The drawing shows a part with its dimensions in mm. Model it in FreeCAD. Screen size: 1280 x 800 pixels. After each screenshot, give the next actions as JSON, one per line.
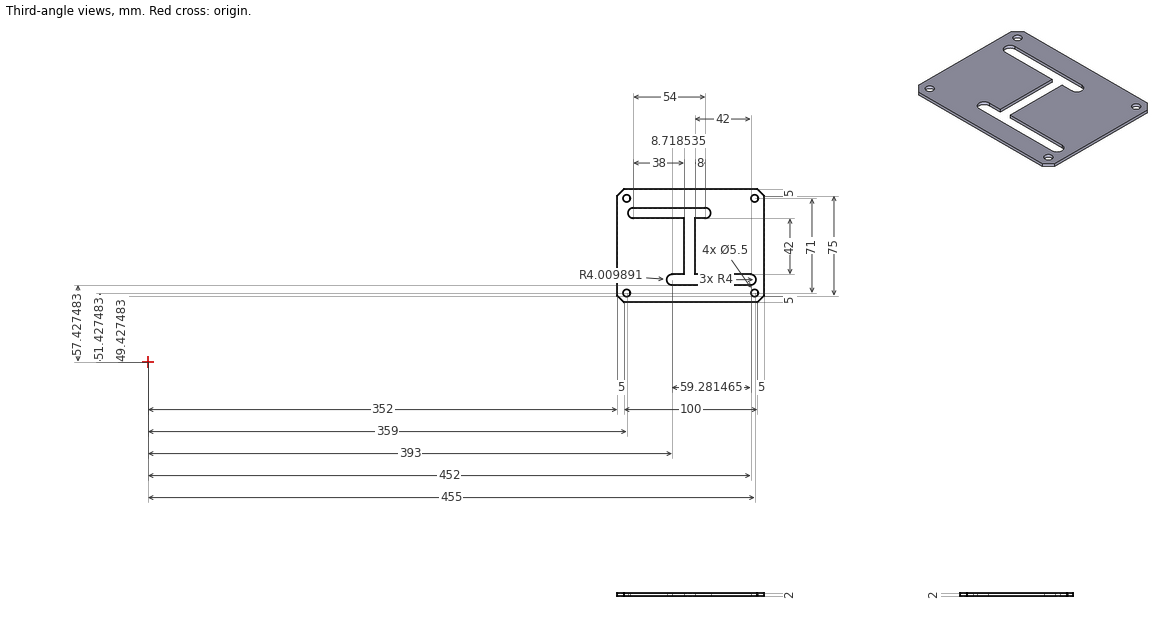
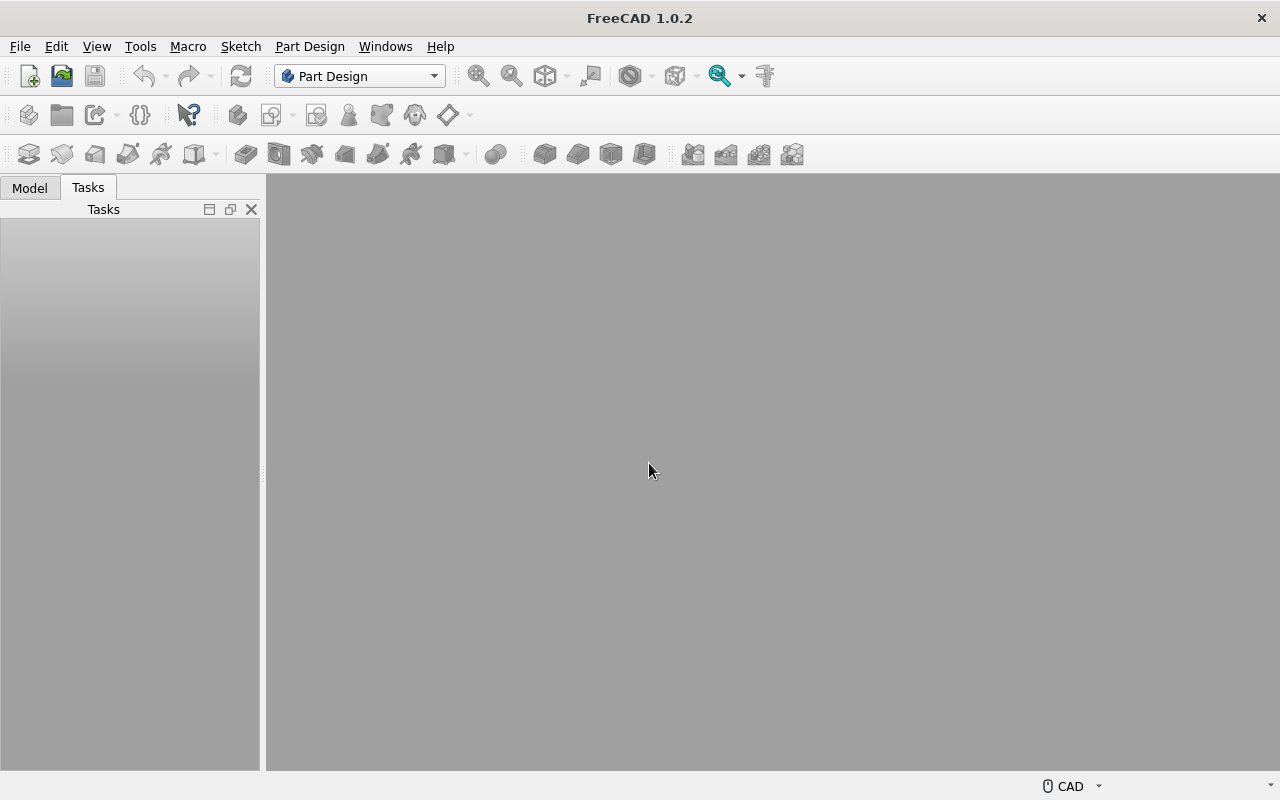
{"action": "left_click", "coordinate": [29, 76]}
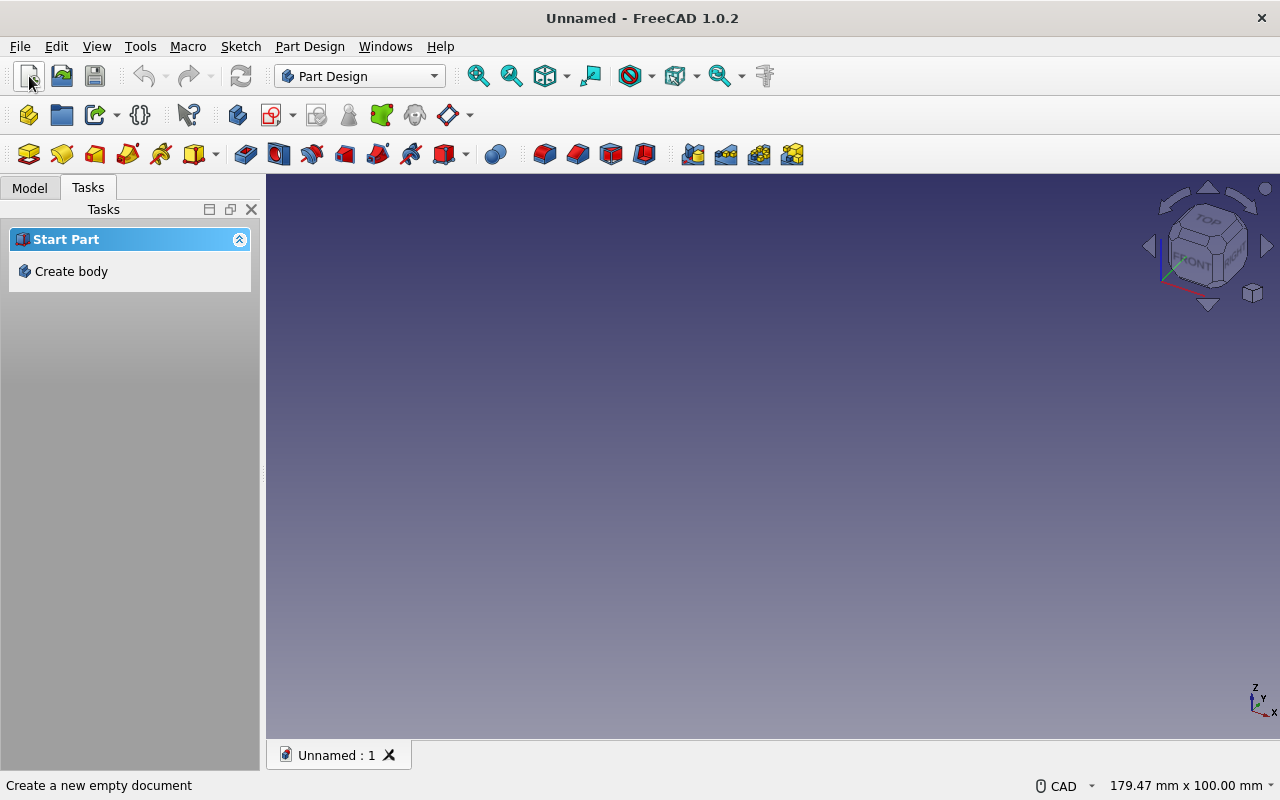
{"action": "left_click", "coordinate": [270, 116]}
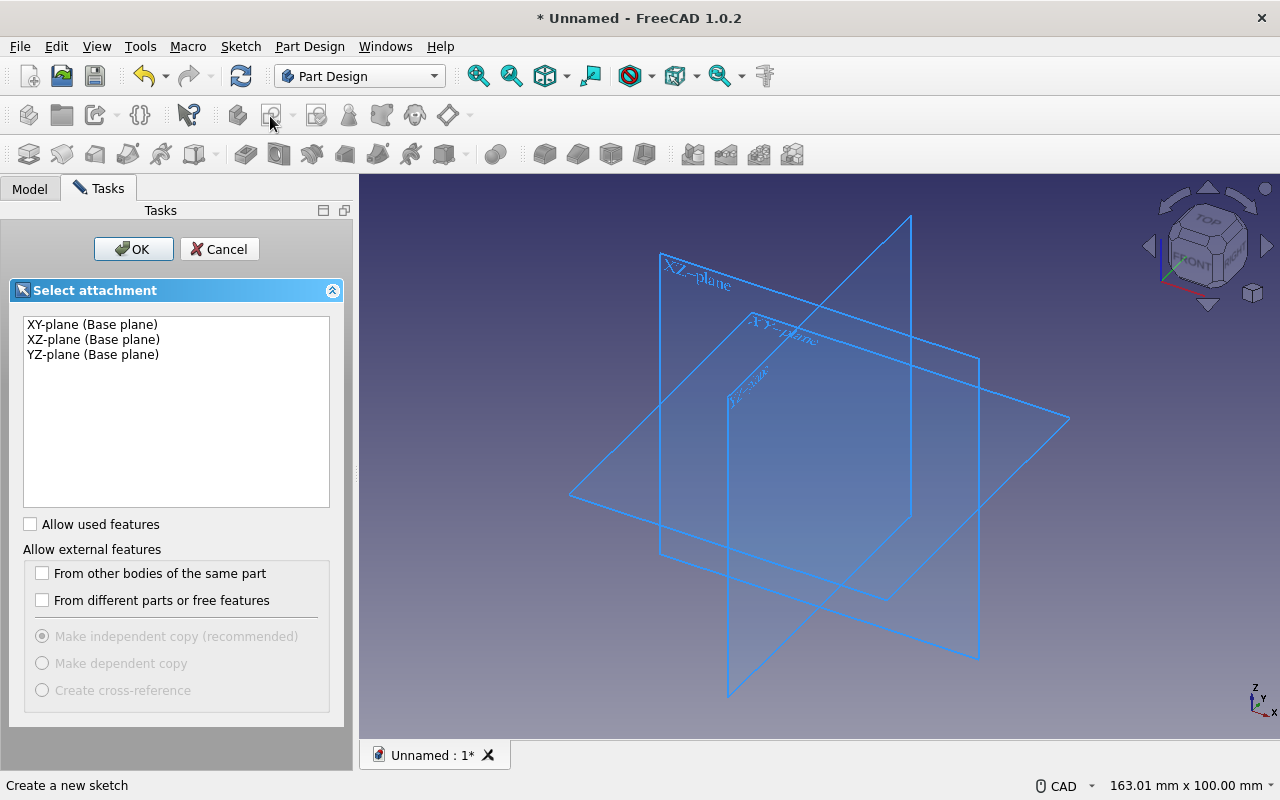
{"action": "left_click", "coordinate": [84, 324]}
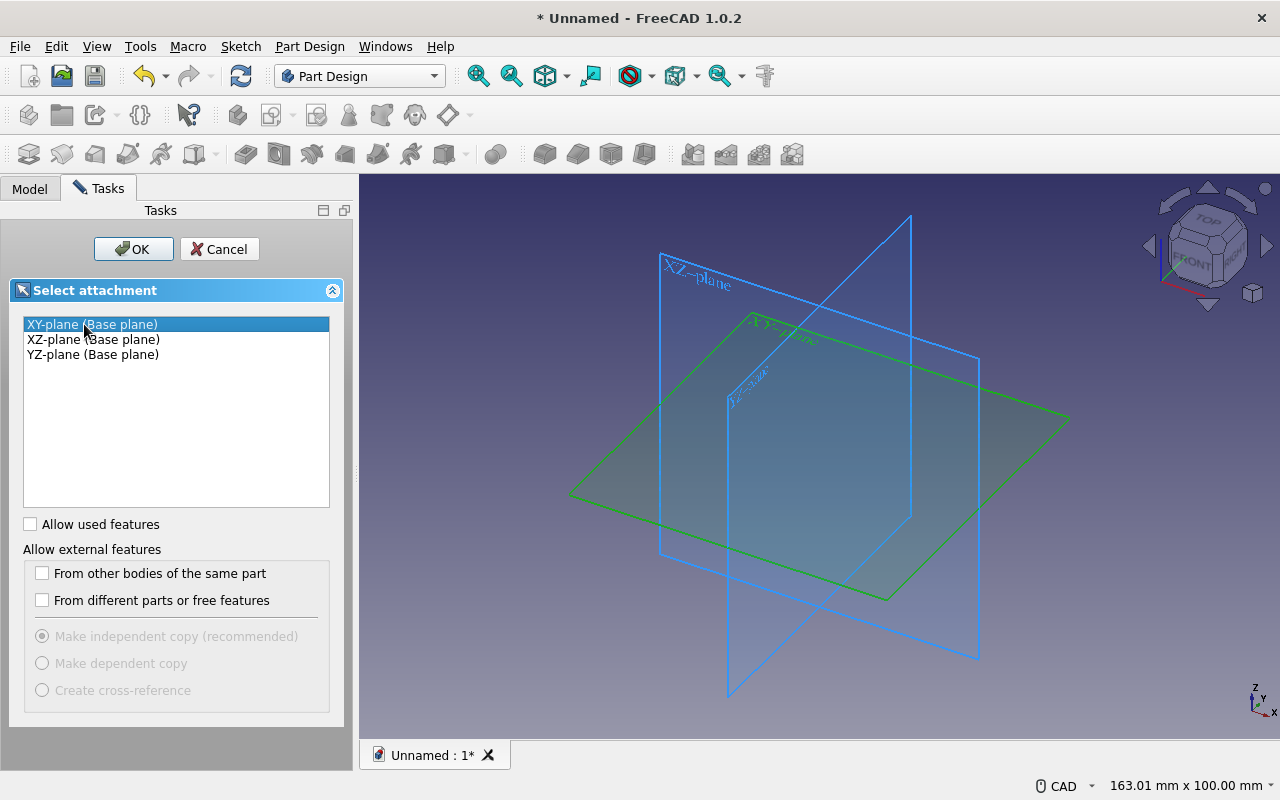
{"action": "left_click", "coordinate": [134, 249]}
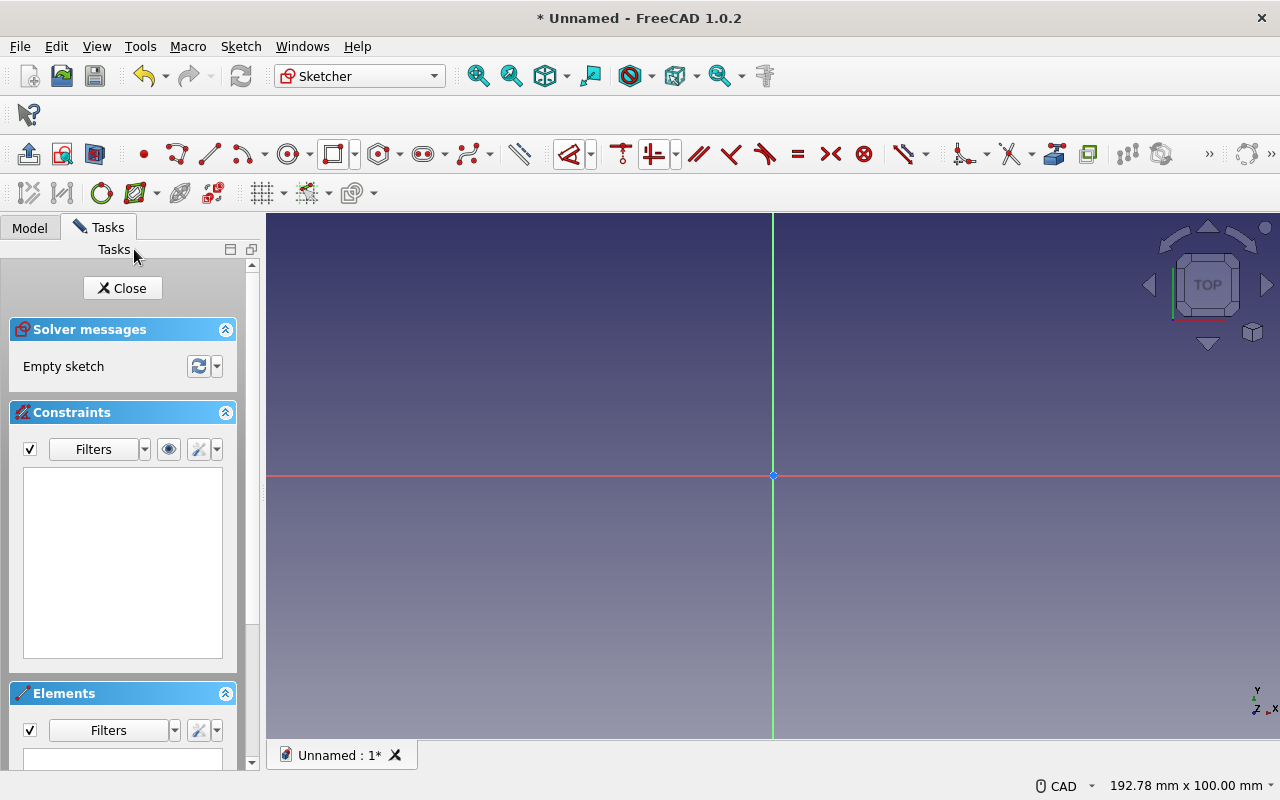
{"action": "scroll", "coordinate": [704, 476], "scroll_direction": "down", "scroll_amount": 5}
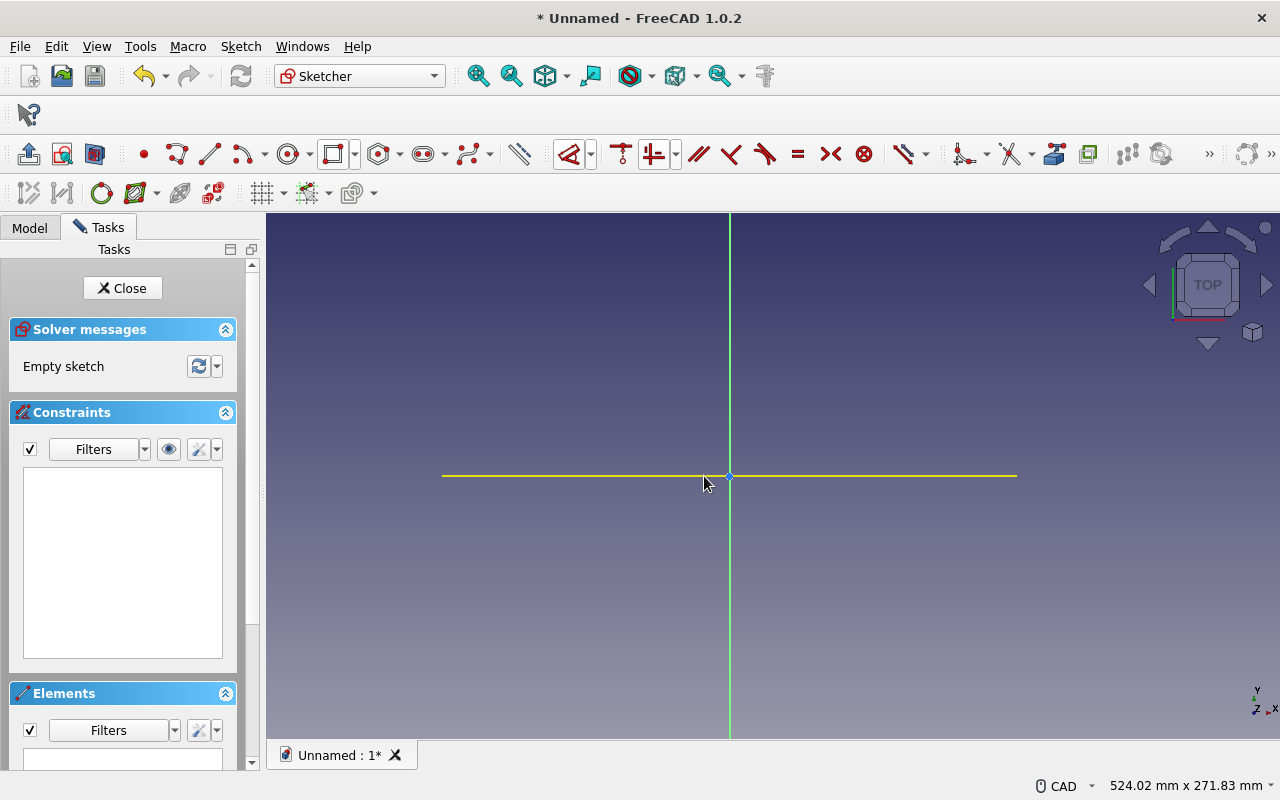
{"action": "scroll", "coordinate": [704, 476], "scroll_direction": "down", "scroll_amount": 5}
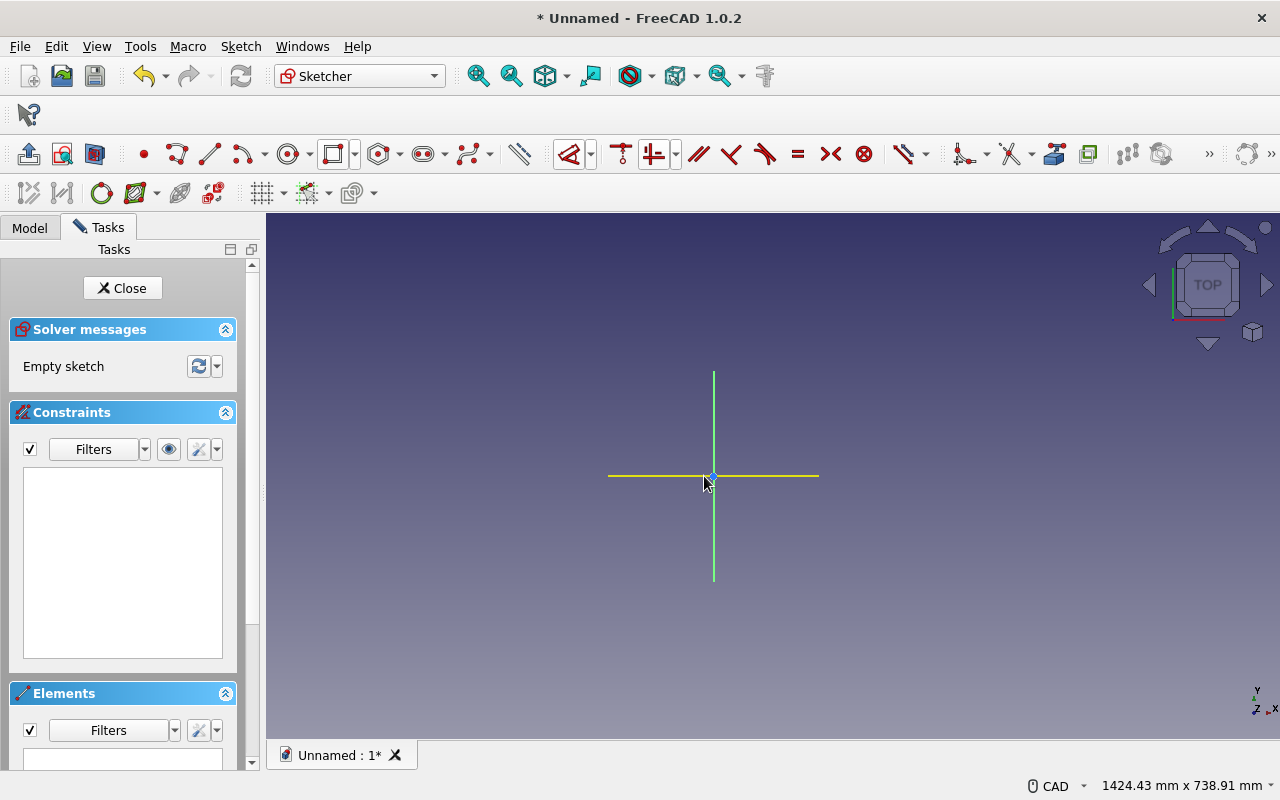
{"action": "scroll", "coordinate": [1063, 402], "scroll_direction": "up", "scroll_amount": 9}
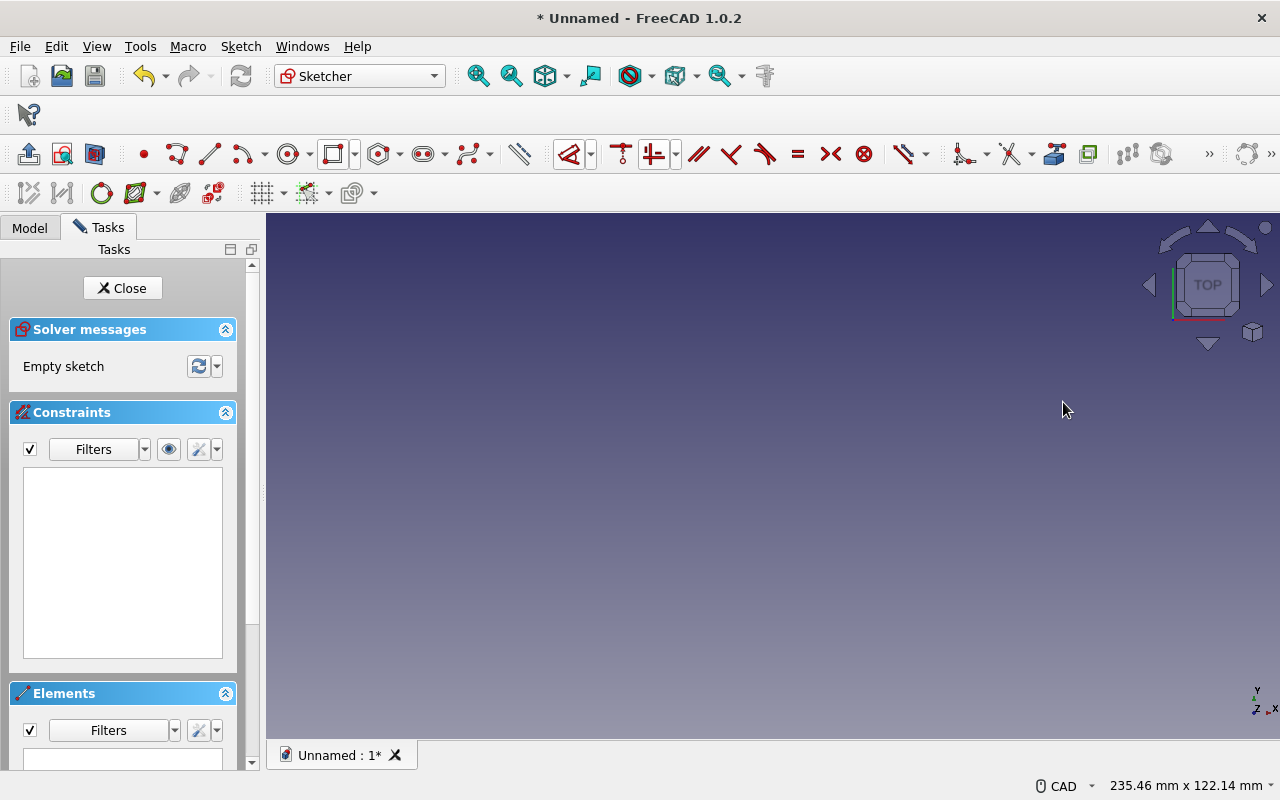
{"action": "left_click", "coordinate": [177, 154]}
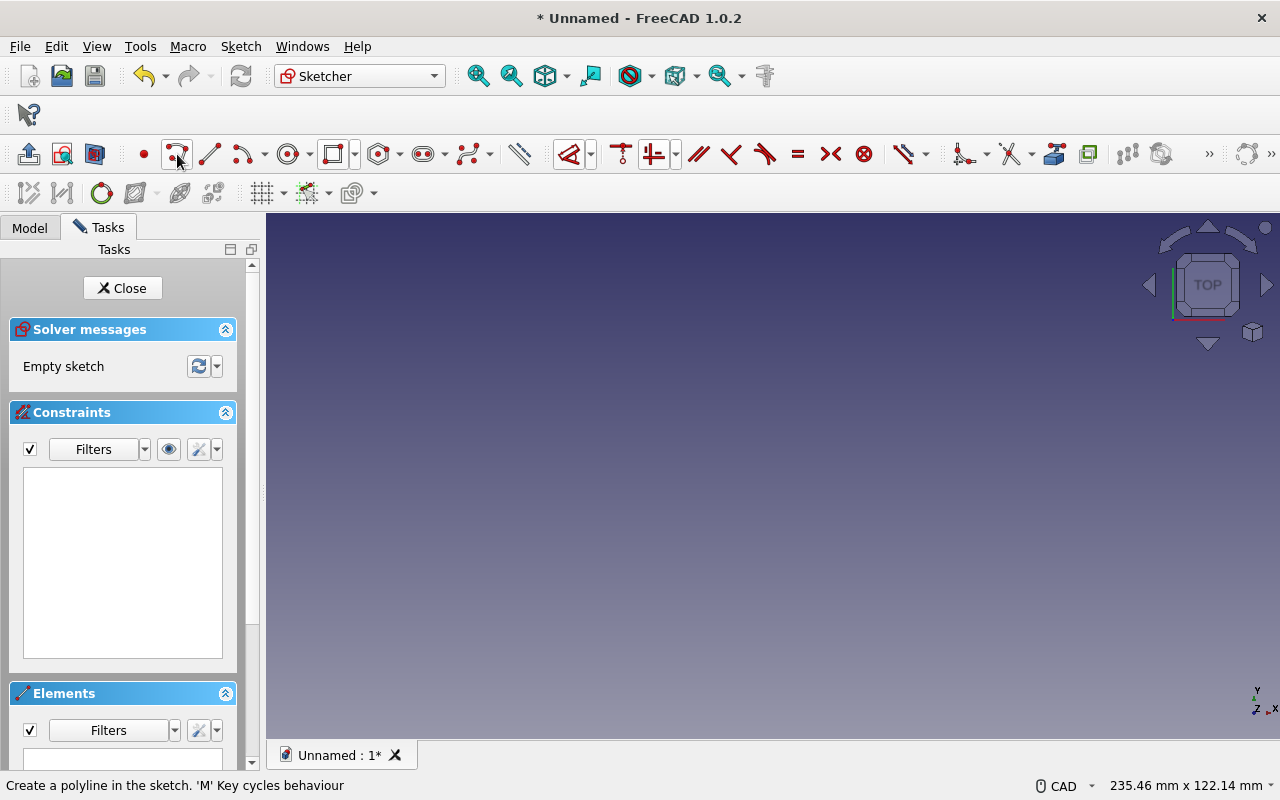
{"action": "left_click", "coordinate": [462, 638]}
{"action": "left_click", "coordinate": [483, 659]}
{"action": "left_click", "coordinate": [914, 659]}
{"action": "left_click", "coordinate": [936, 638]}
{"action": "left_click", "coordinate": [936, 315]}
{"action": "left_click", "coordinate": [914, 293]}
{"action": "left_click", "coordinate": [483, 293]}
{"action": "left_click", "coordinate": [462, 315]}
{"action": "left_click", "coordinate": [462, 639]}
{"action": "key", "text": "Escape"}
{"action": "key", "text": "Escape"}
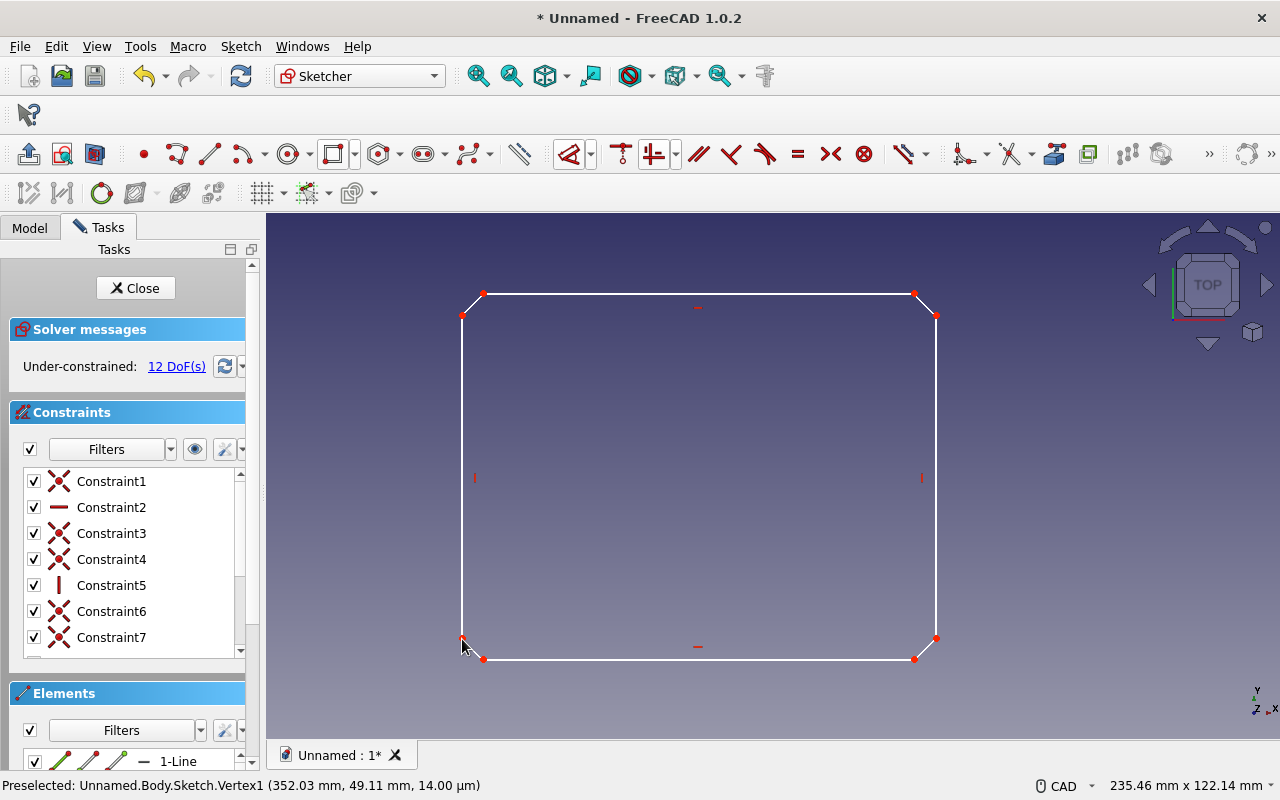
{"action": "left_click", "coordinate": [936, 542]}